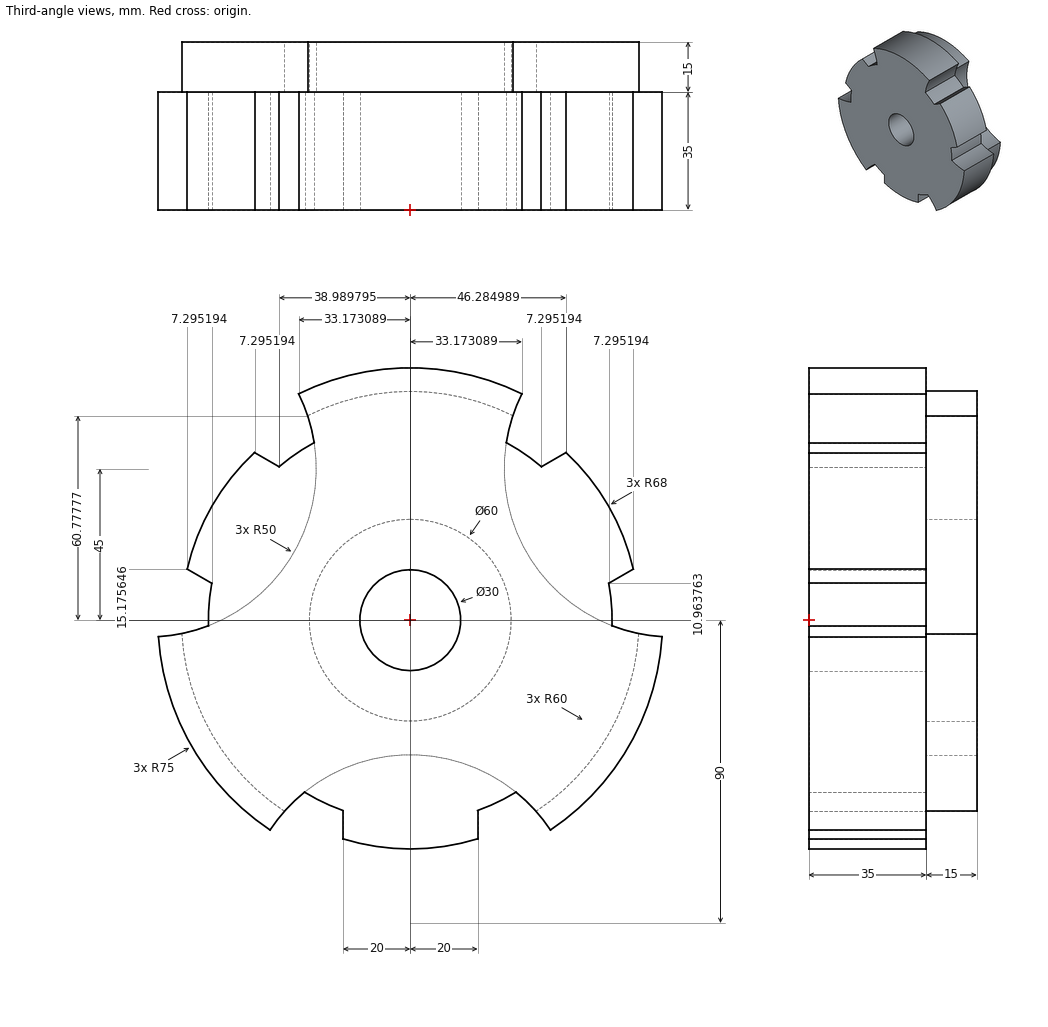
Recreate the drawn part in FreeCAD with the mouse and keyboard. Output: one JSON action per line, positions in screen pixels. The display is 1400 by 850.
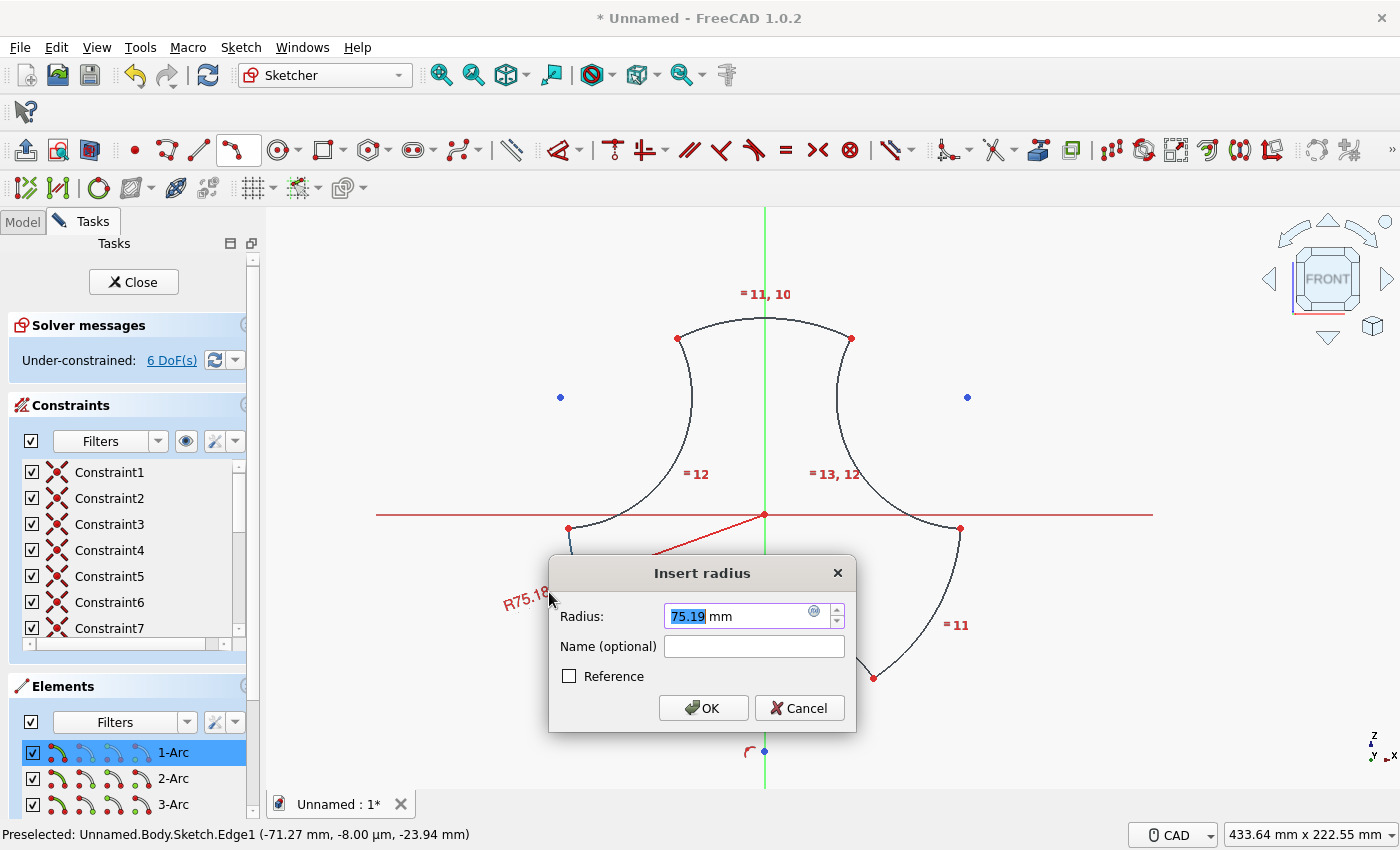
{"action": "type", "text": "75"}
{"action": "key", "text": "Return"}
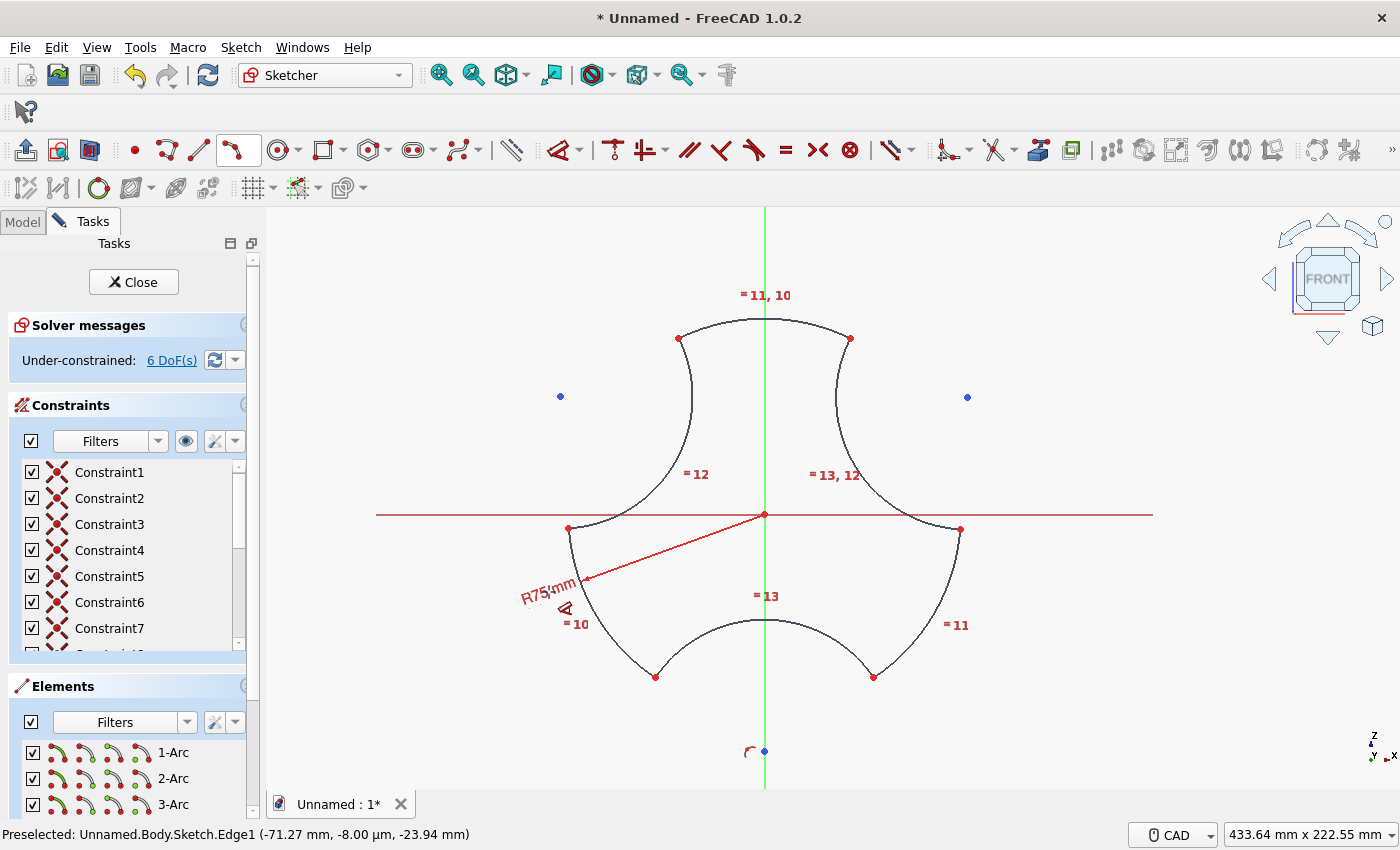
{"action": "left_click", "coordinate": [641, 502]}
{"action": "left_click", "coordinate": [711, 464]}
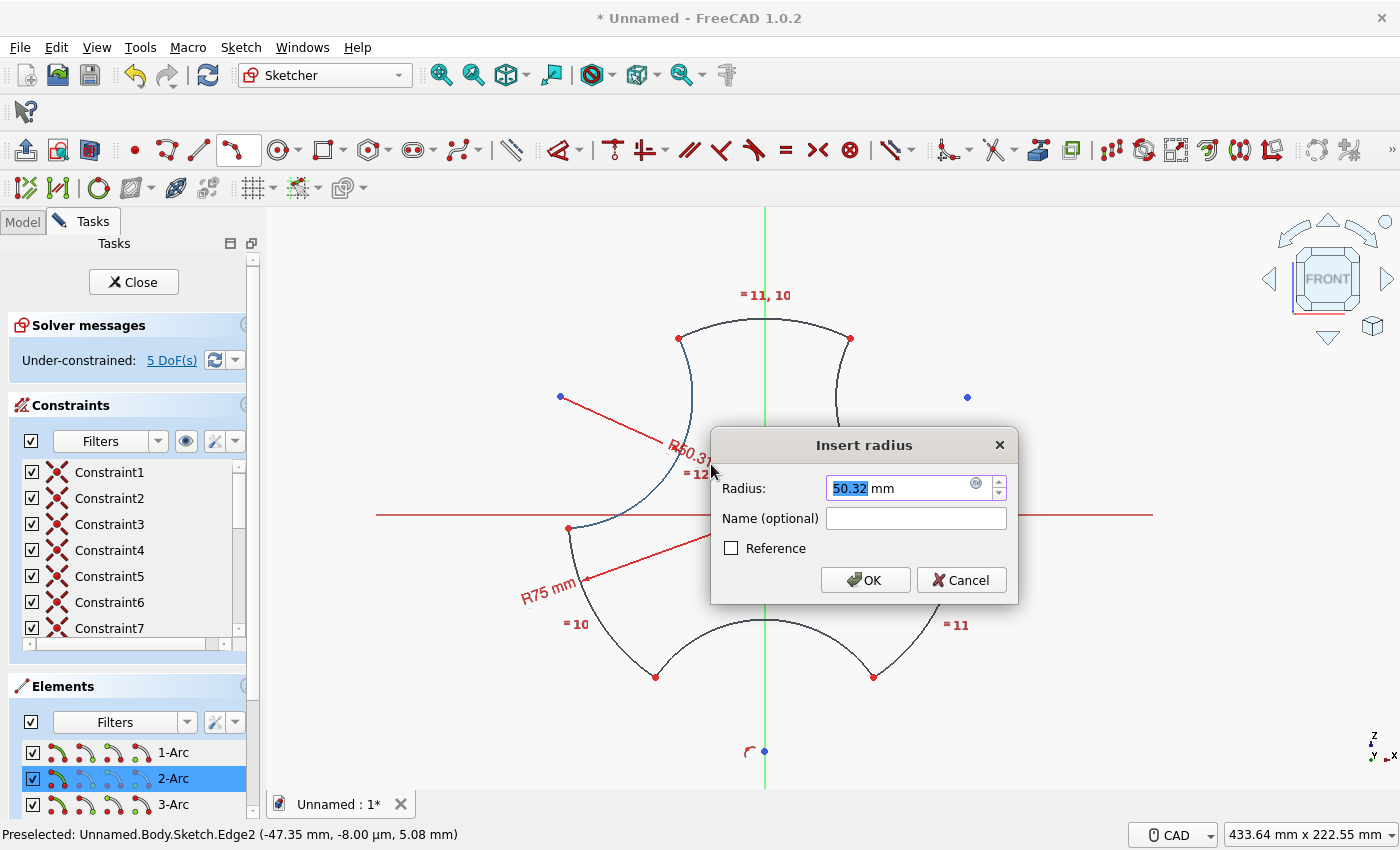
{"action": "type", "text": "50"}
{"action": "key", "text": "Return"}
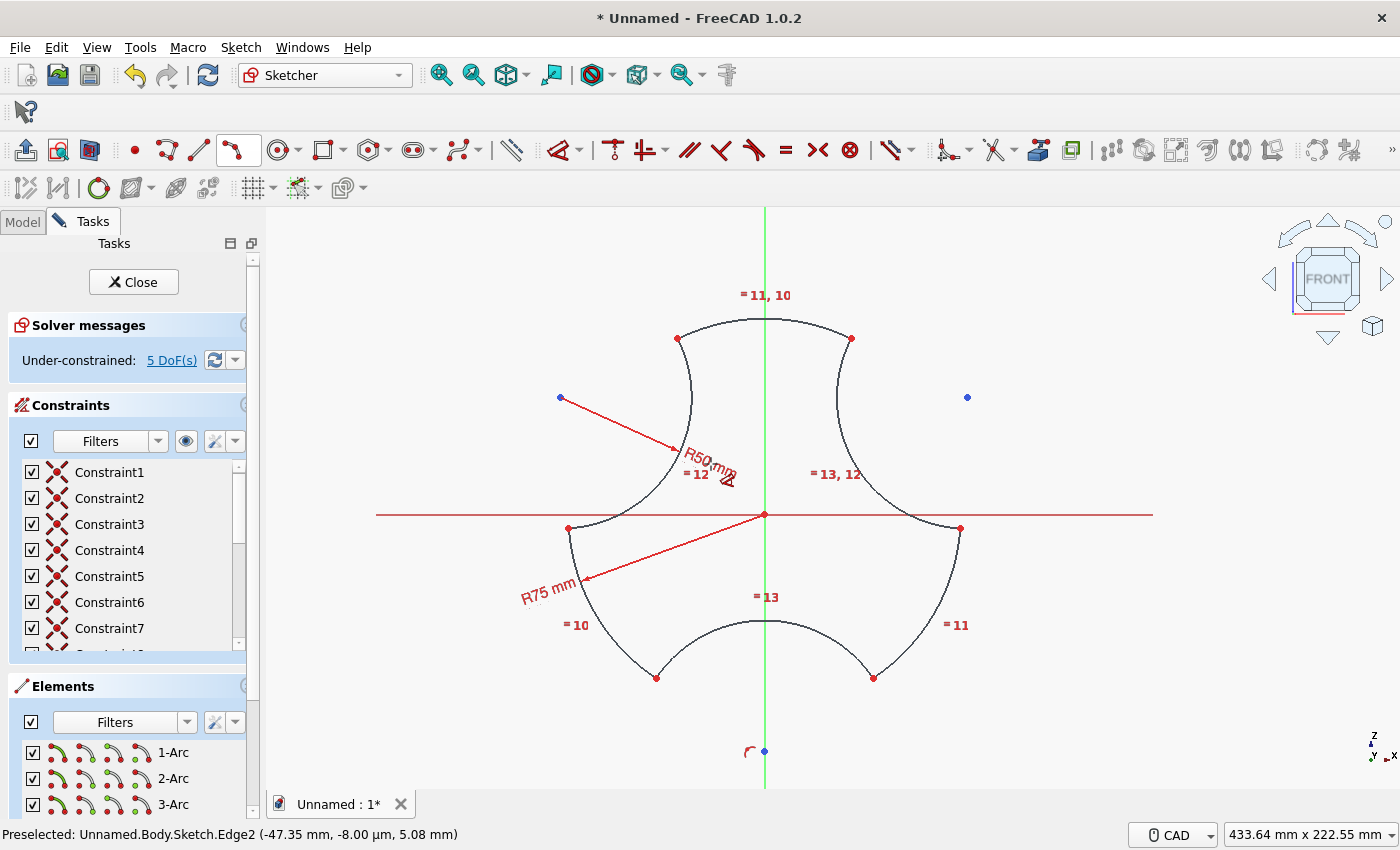
{"action": "left_click", "coordinate": [561, 398]}
{"action": "left_click", "coordinate": [527, 456]}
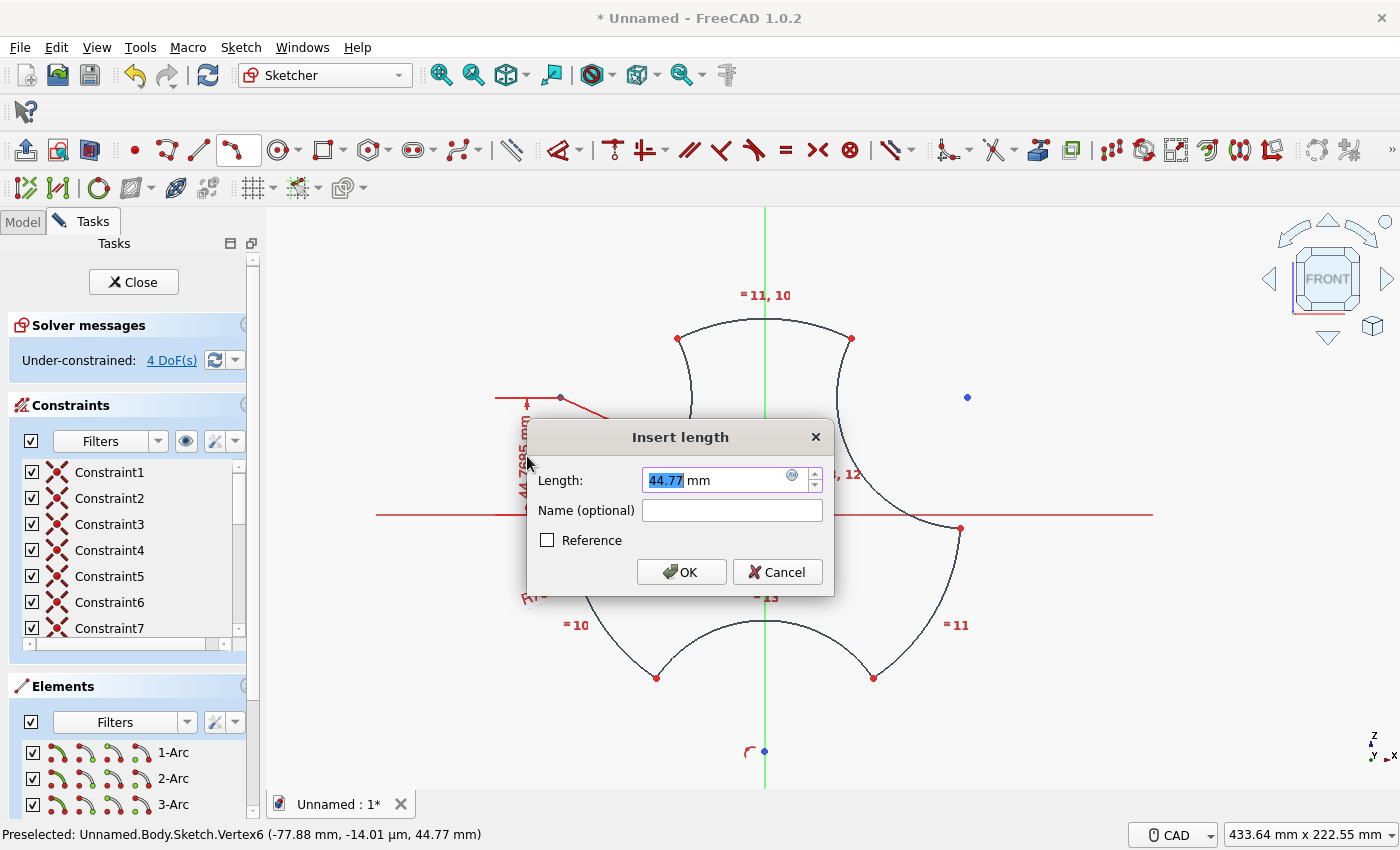
{"action": "type", "text": "45"}
{"action": "key", "text": "Return"}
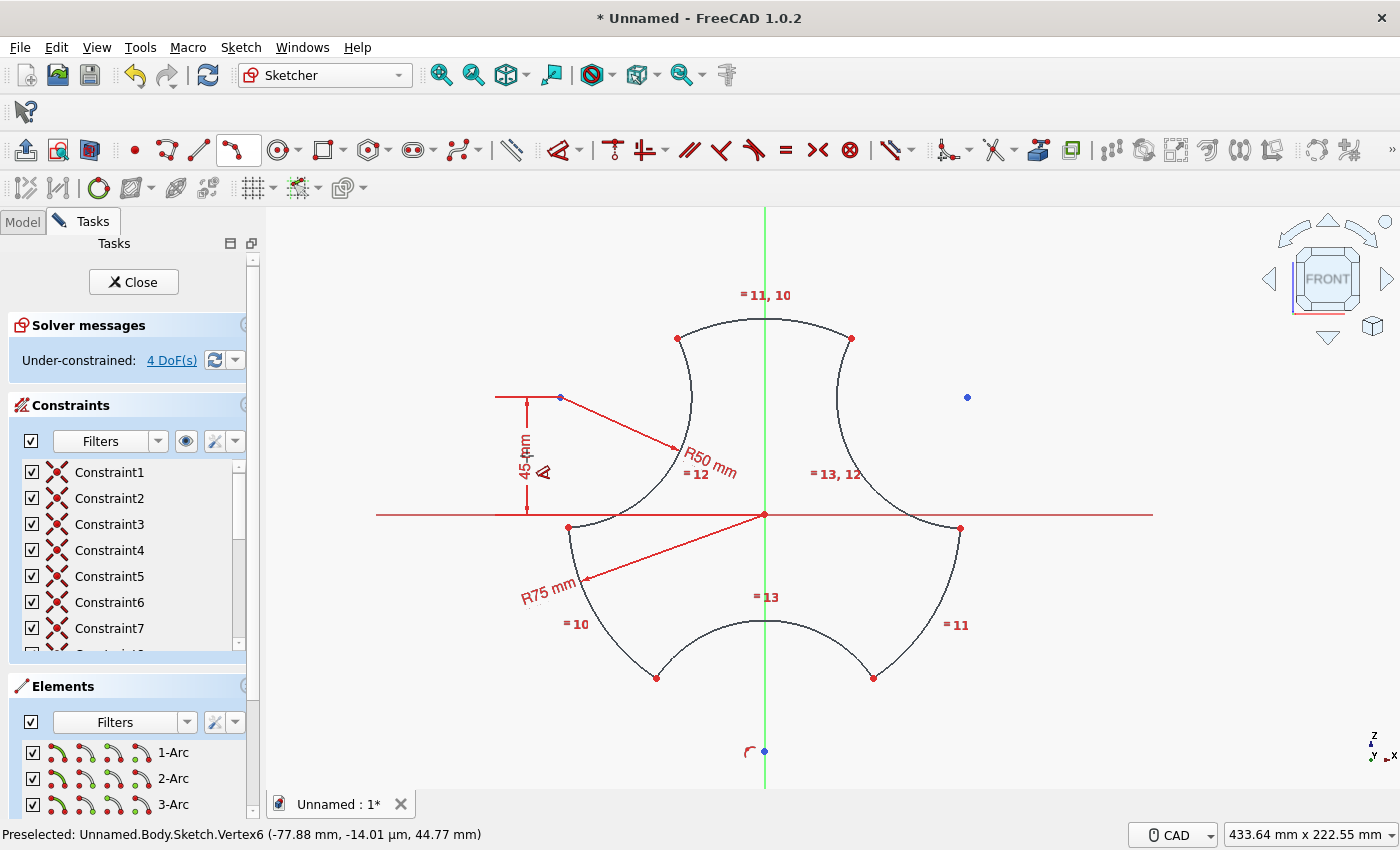
{"action": "left_click", "coordinate": [968, 398]}
{"action": "left_click", "coordinate": [1002, 456]}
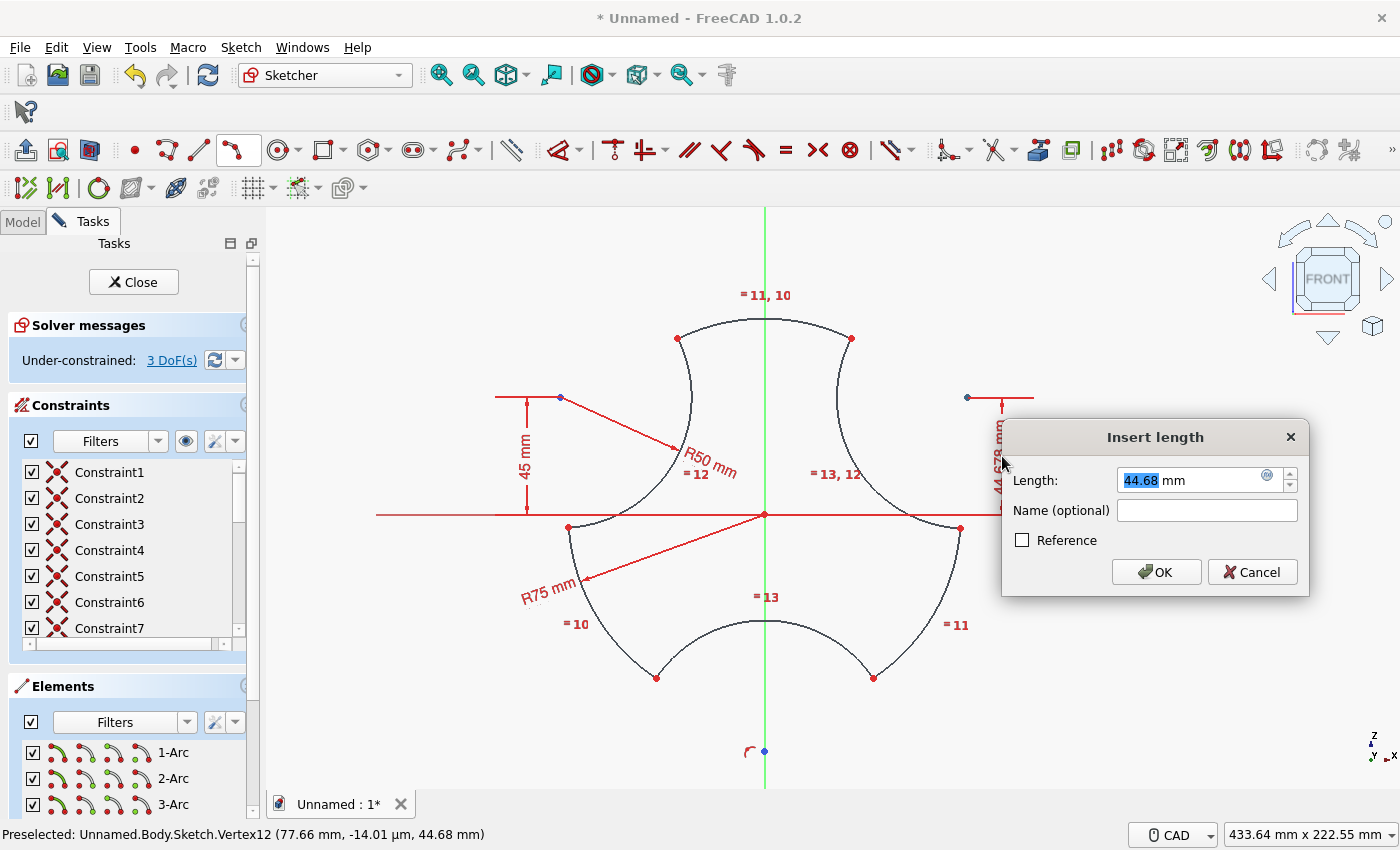
{"action": "type", "text": "45"}
{"action": "key", "text": "Return"}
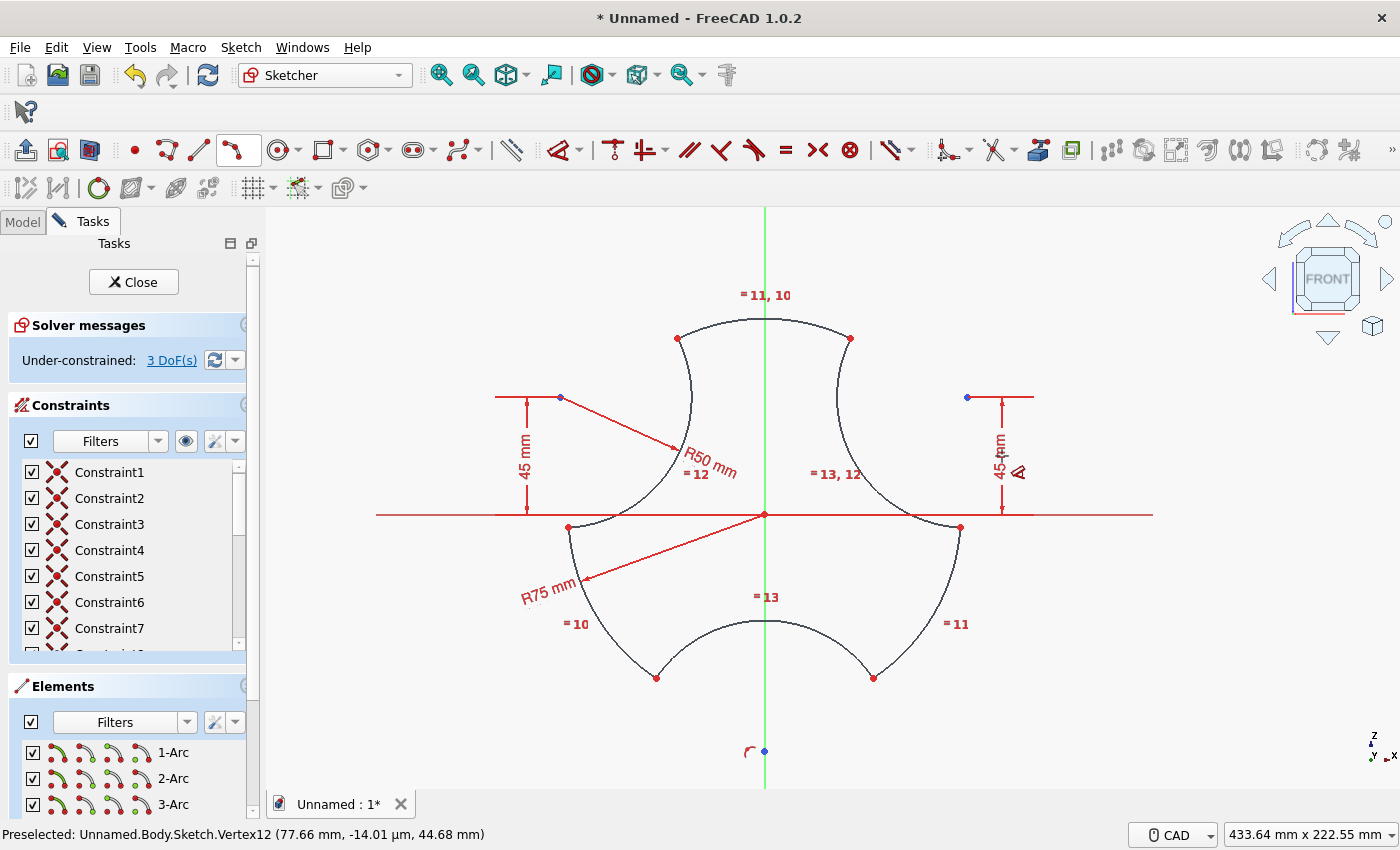
{"action": "left_click", "coordinate": [765, 751]}
{"action": "left_click", "coordinate": [799, 579]}